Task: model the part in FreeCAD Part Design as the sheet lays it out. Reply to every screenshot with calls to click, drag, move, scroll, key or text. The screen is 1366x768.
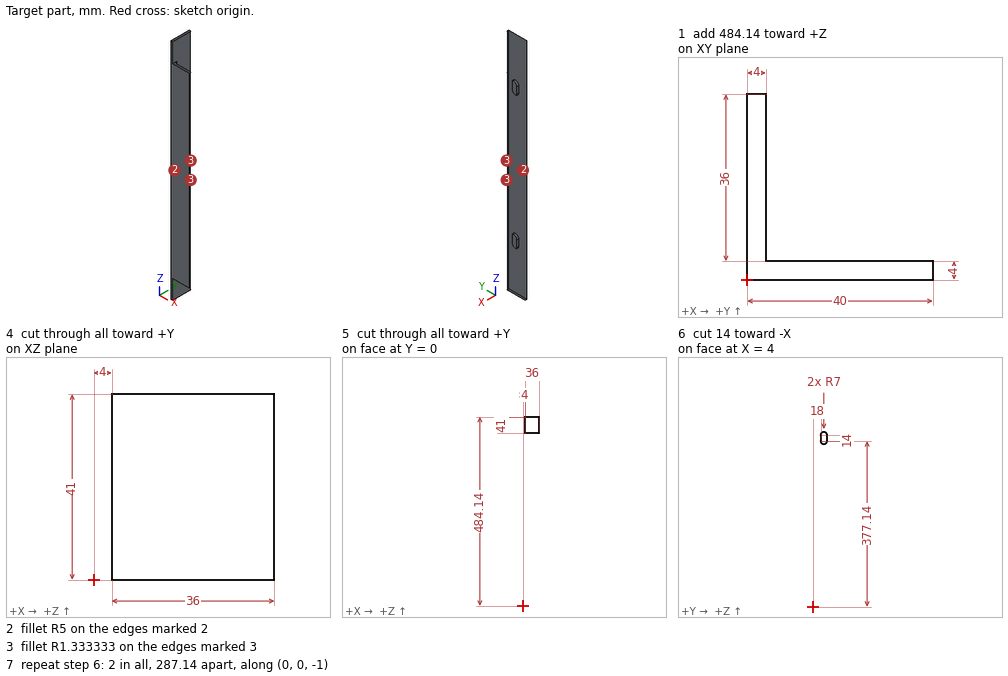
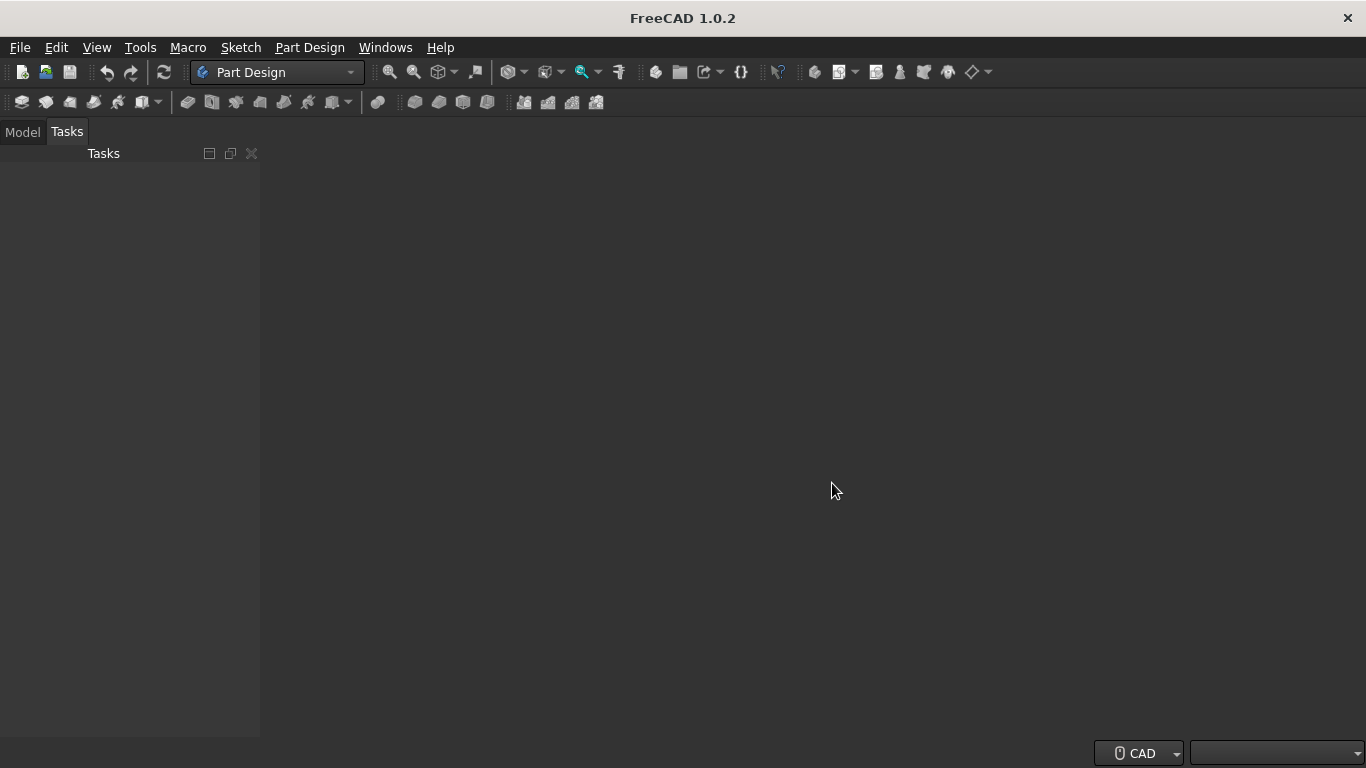
click(22, 72)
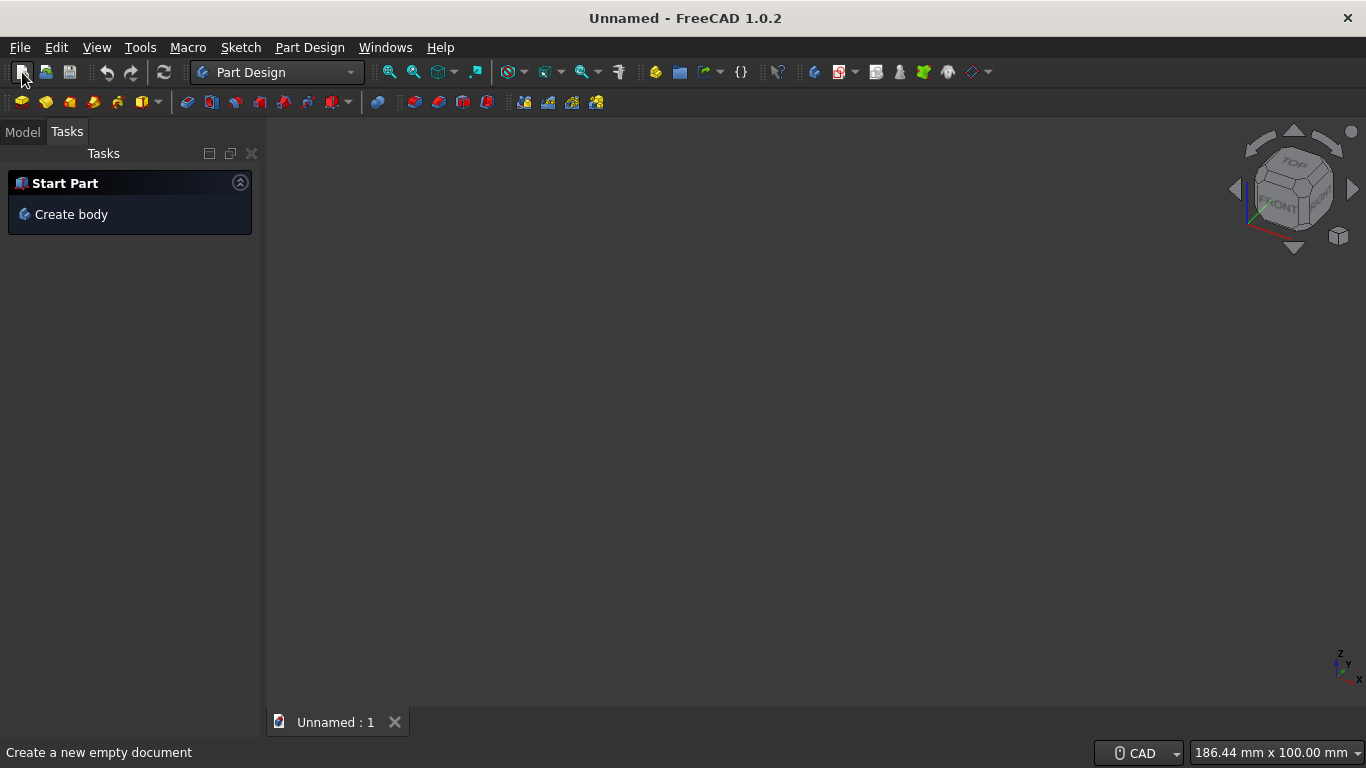
click(840, 72)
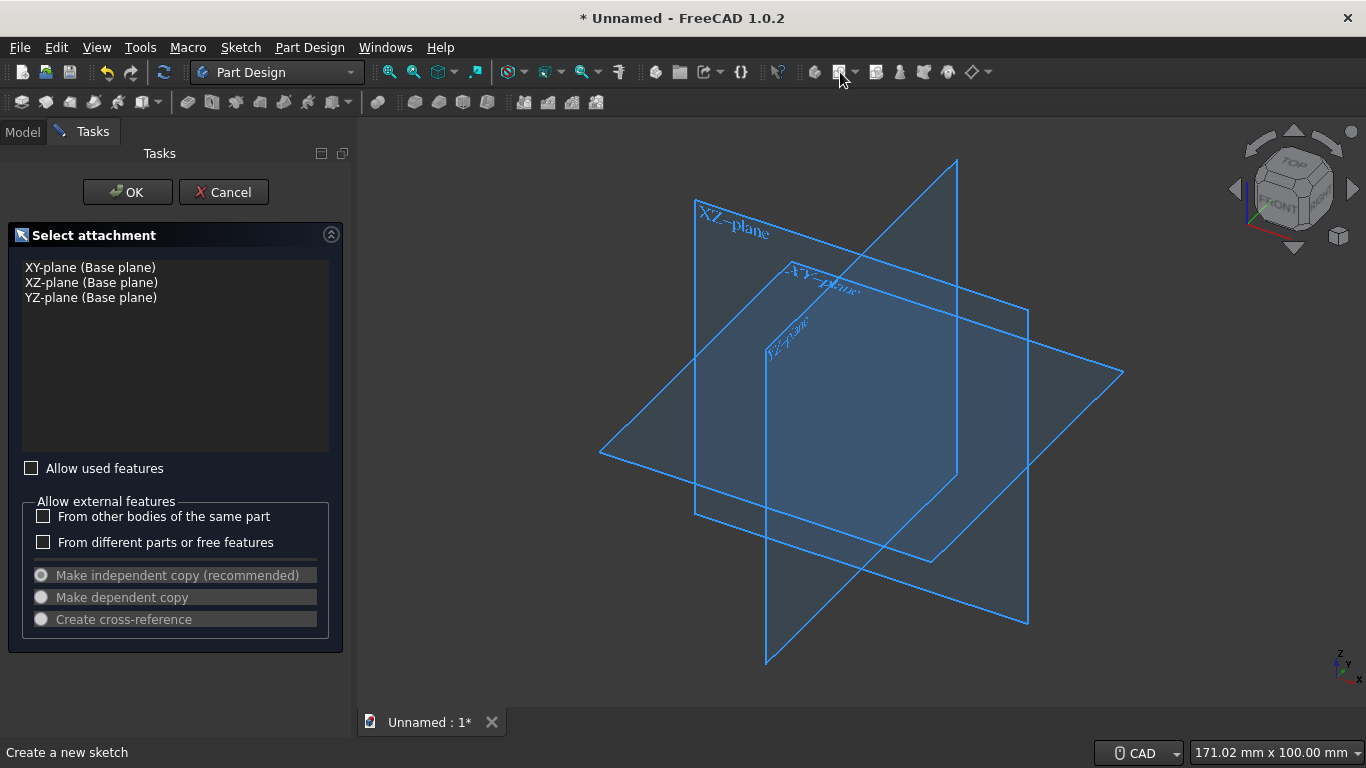
click(82, 268)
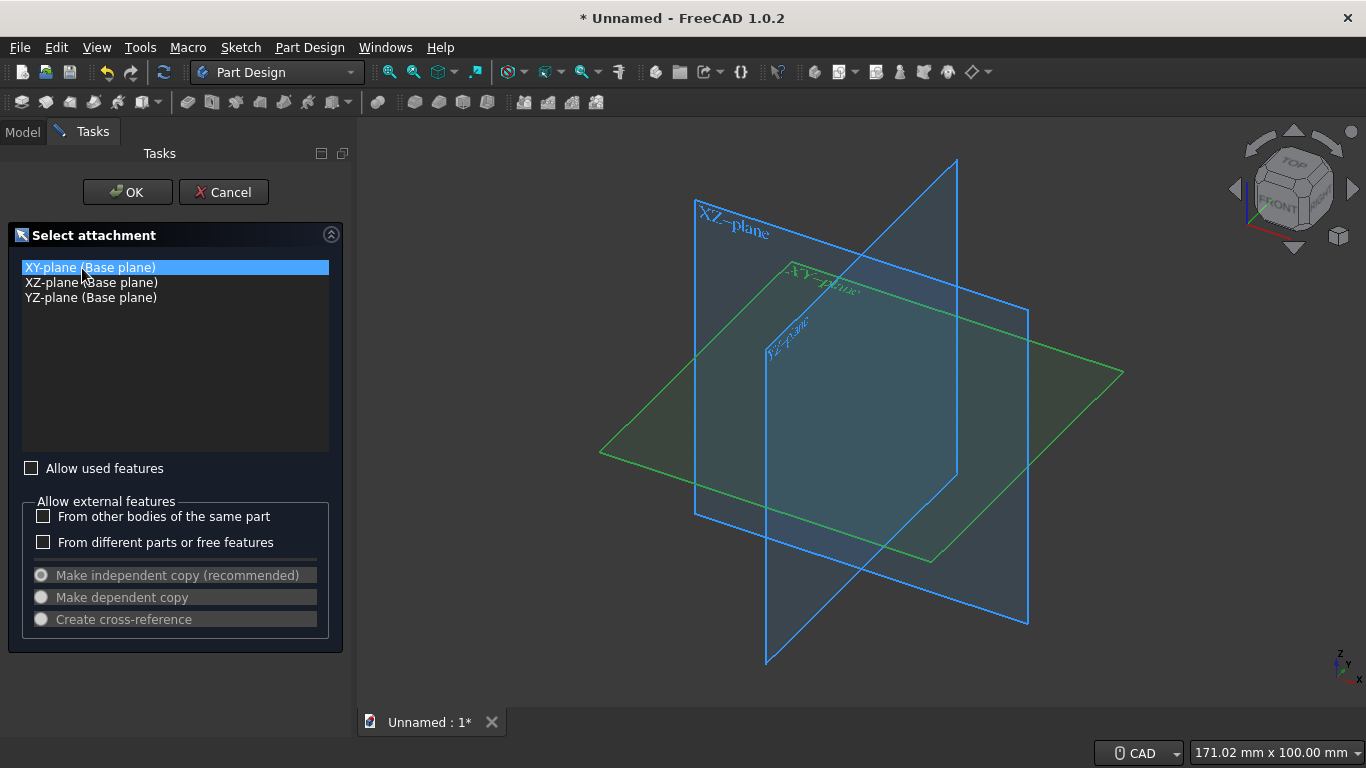
click(128, 192)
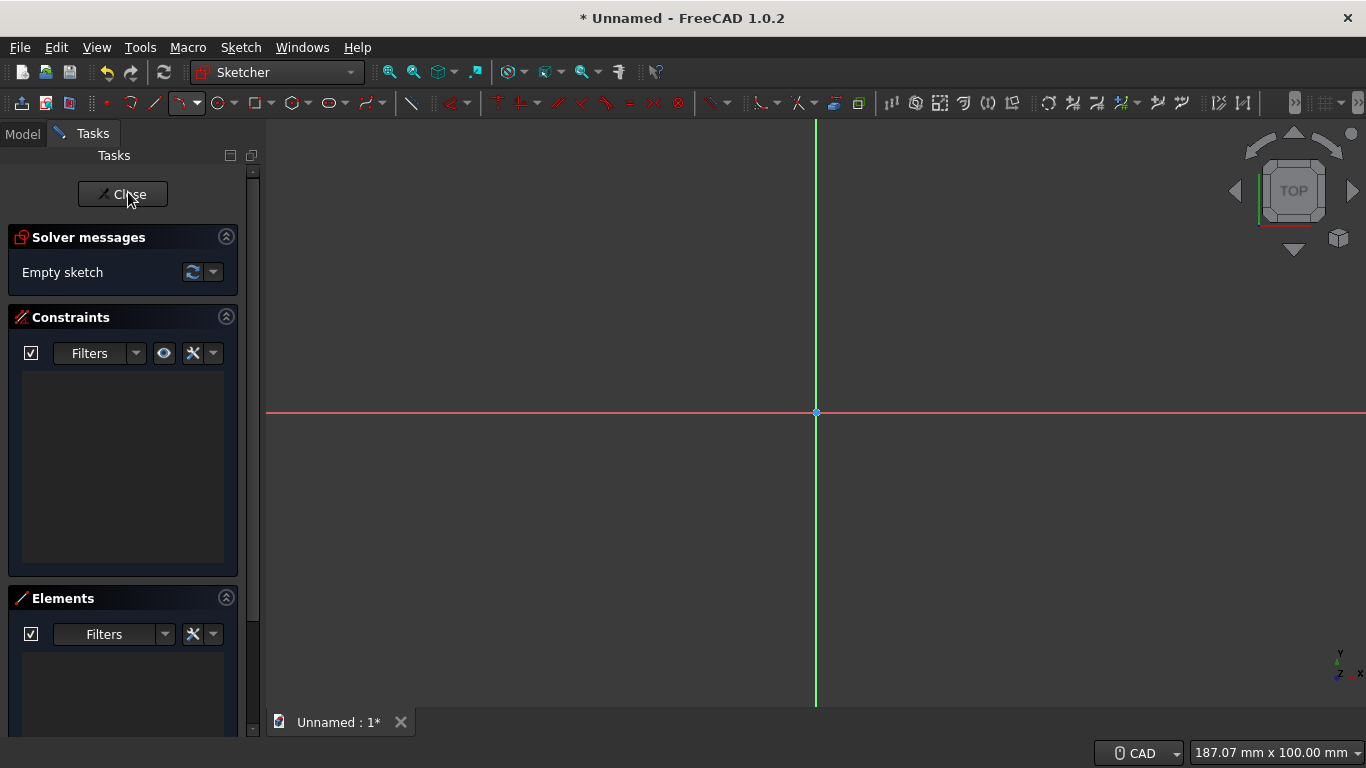
scroll(1201, 147, up, 2)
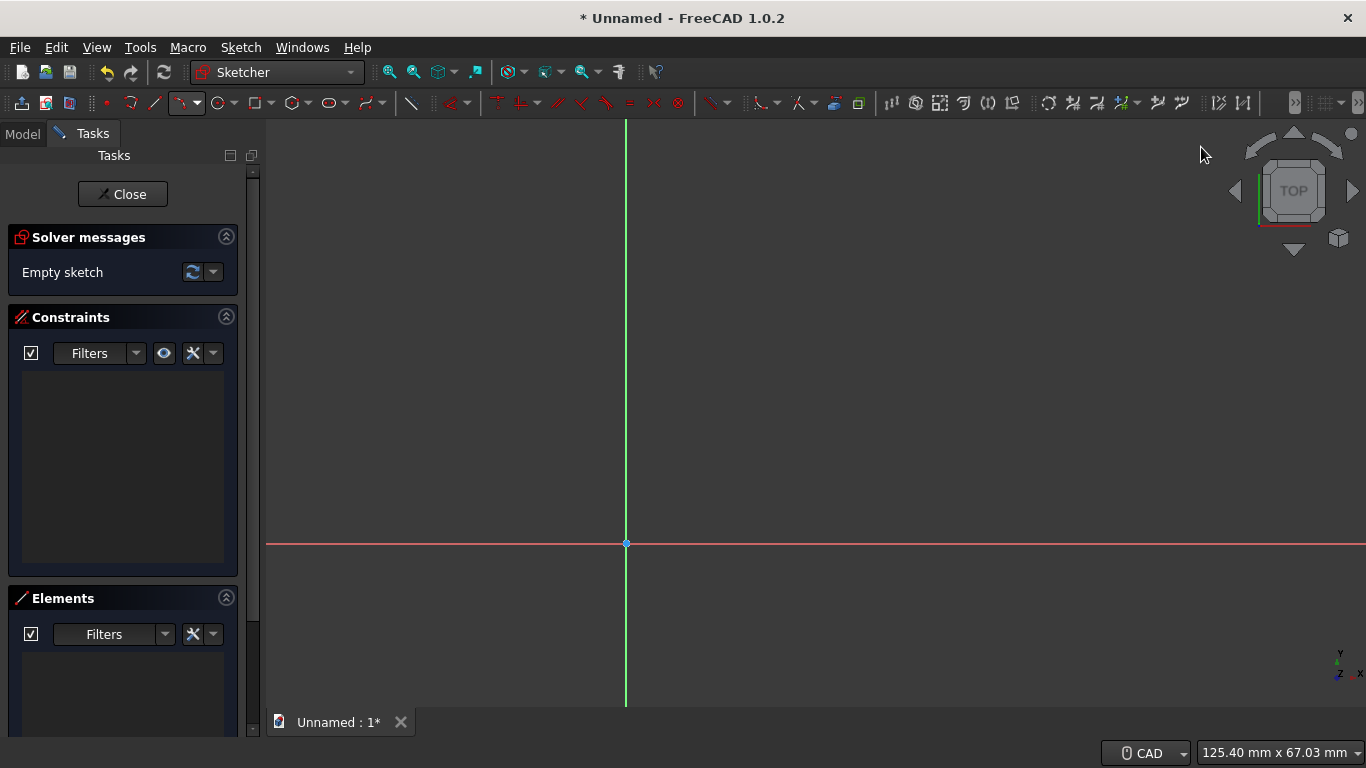
click(132, 104)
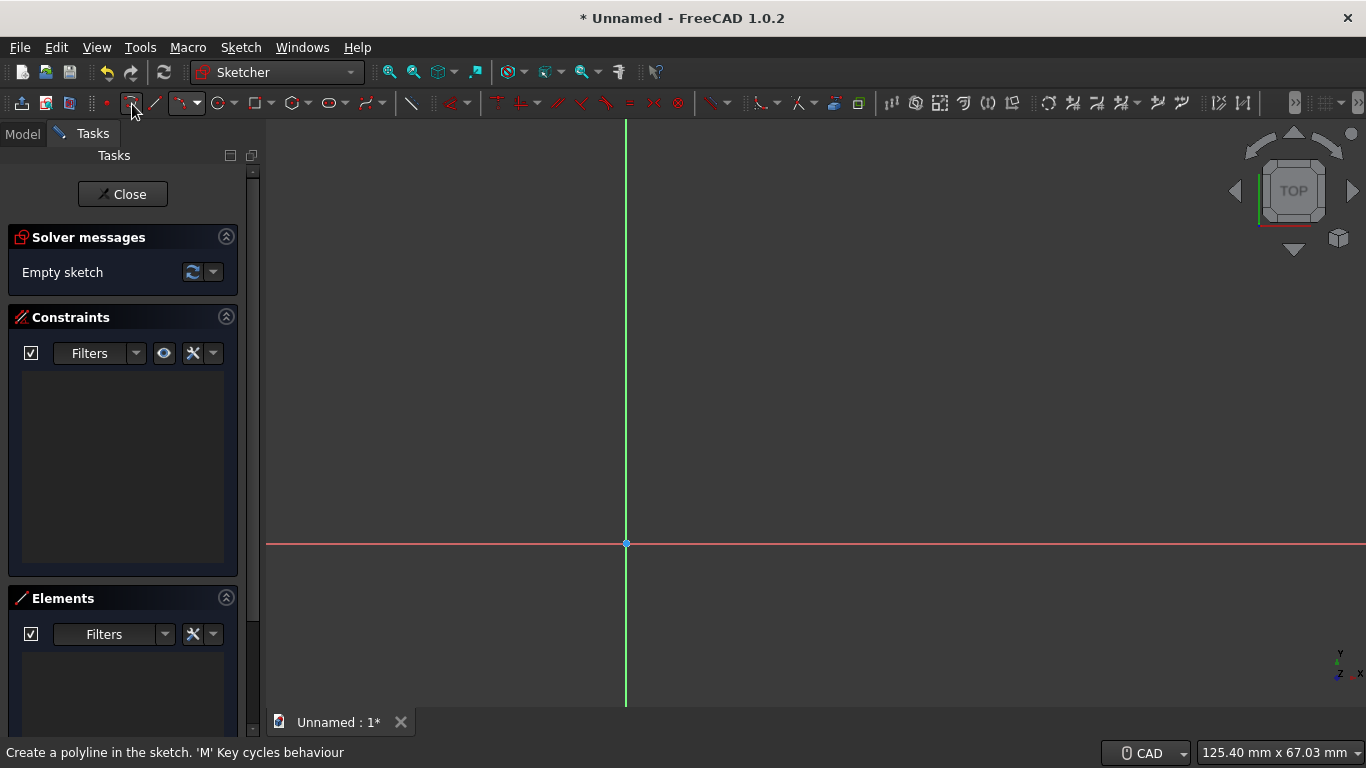
click(626, 544)
click(977, 535)
click(977, 509)
click(661, 509)
click(661, 193)
click(635, 193)
click(626, 544)
key(Escape)
key(Escape)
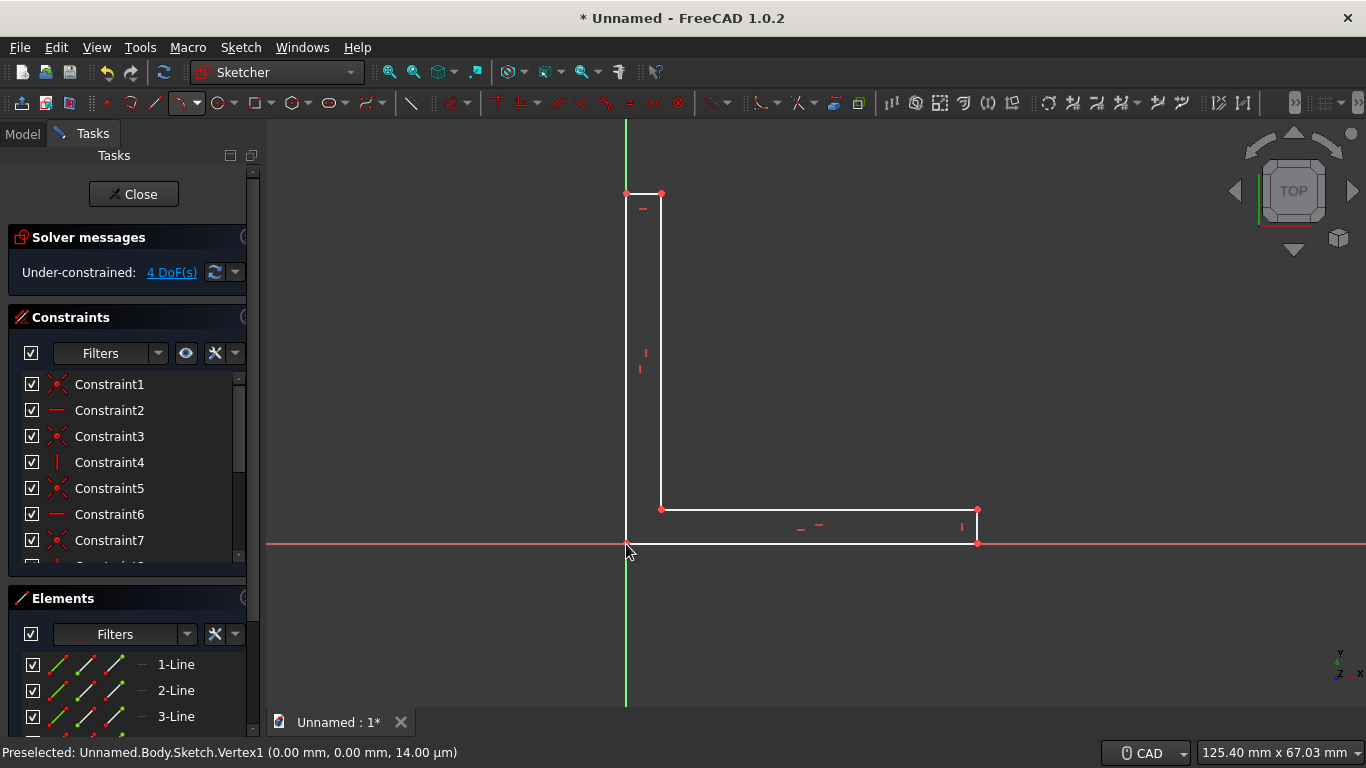
scroll(977, 534, up, 2)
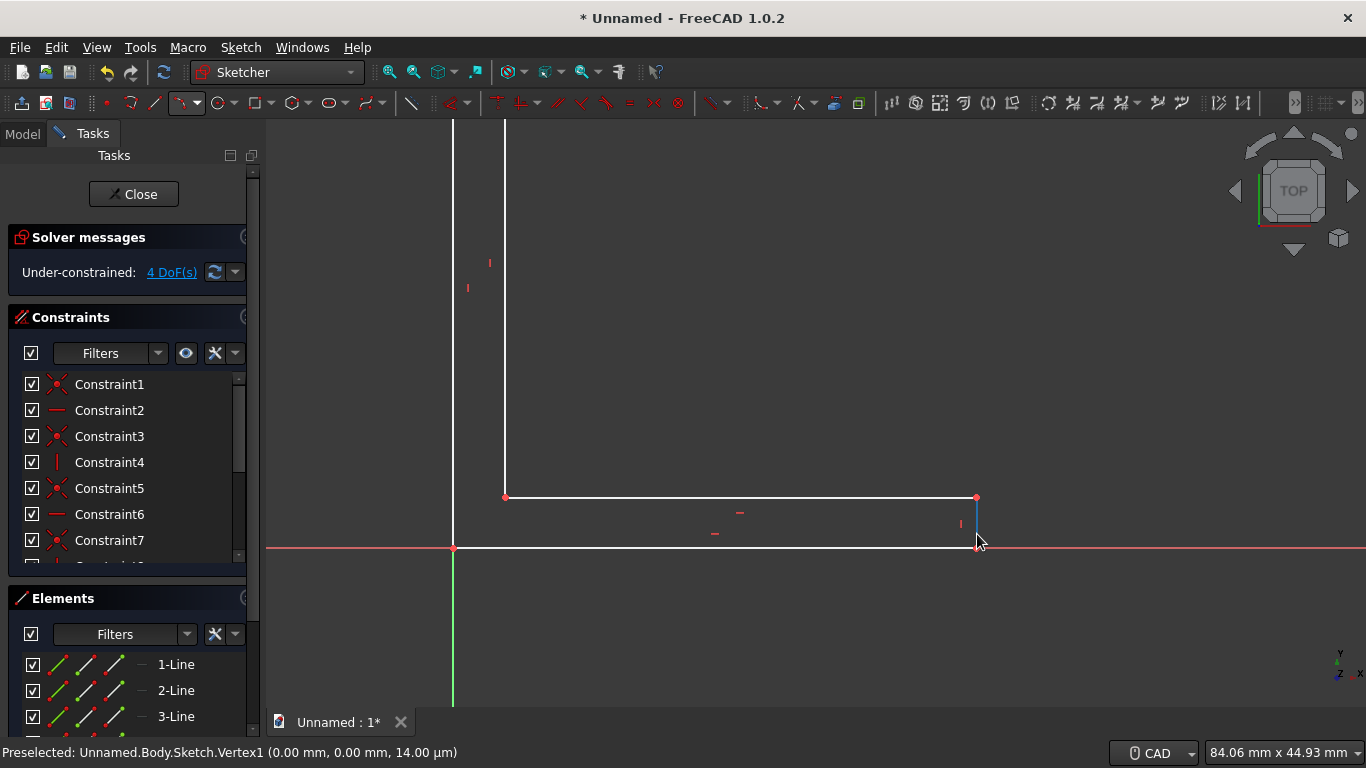
click(977, 533)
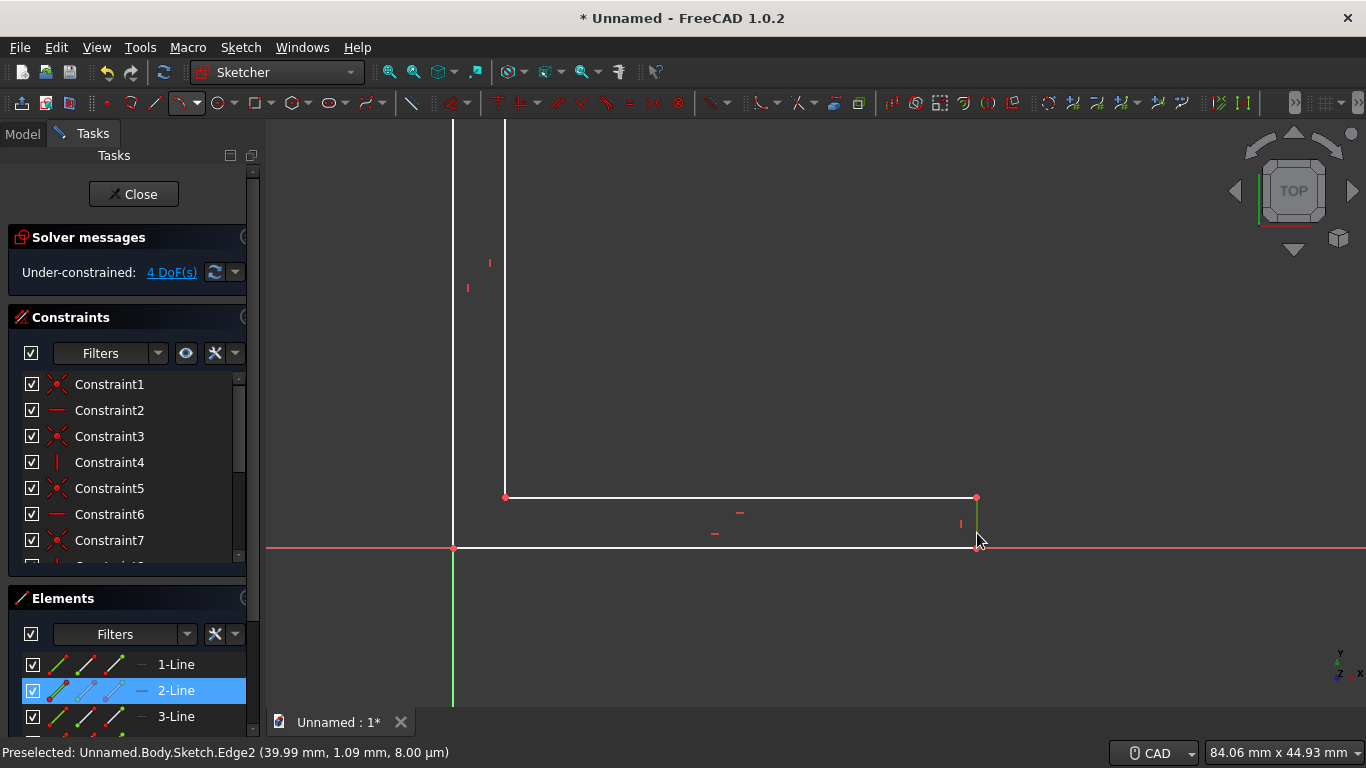
click(470, 104)